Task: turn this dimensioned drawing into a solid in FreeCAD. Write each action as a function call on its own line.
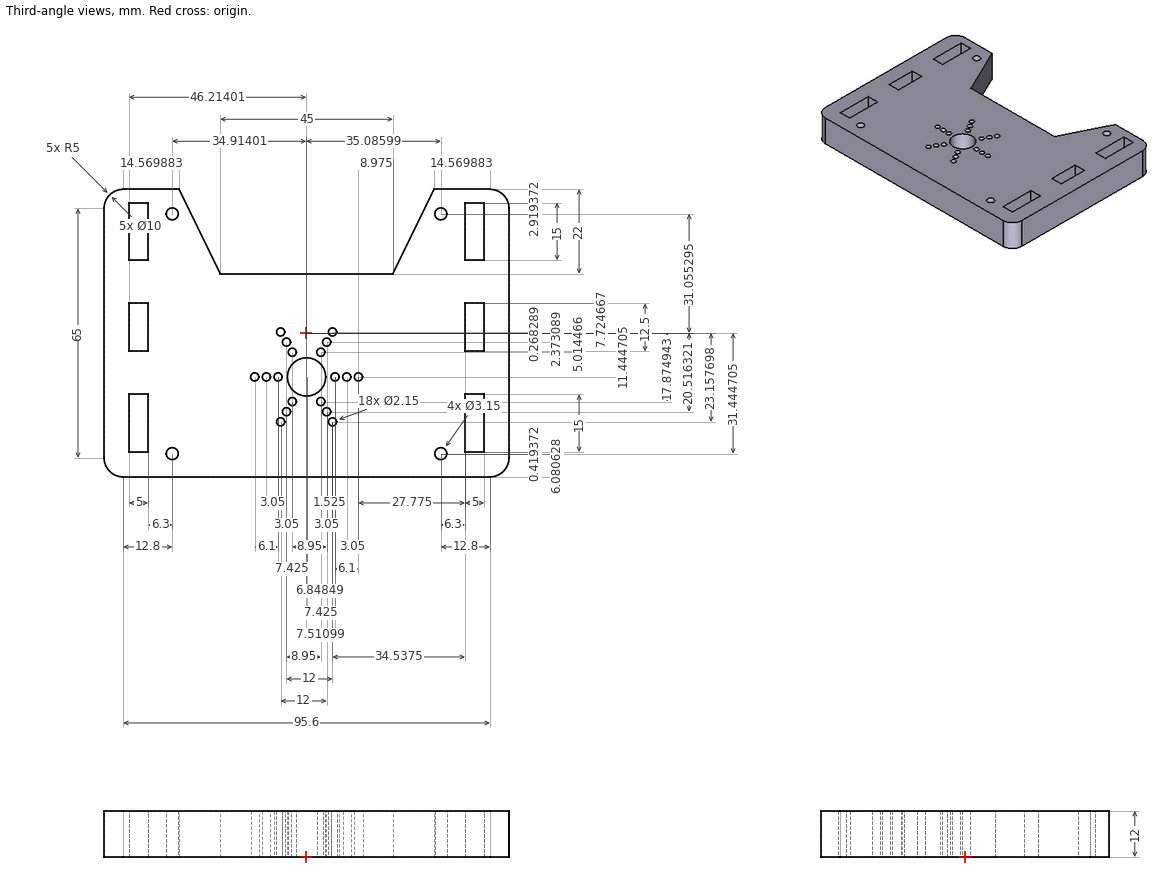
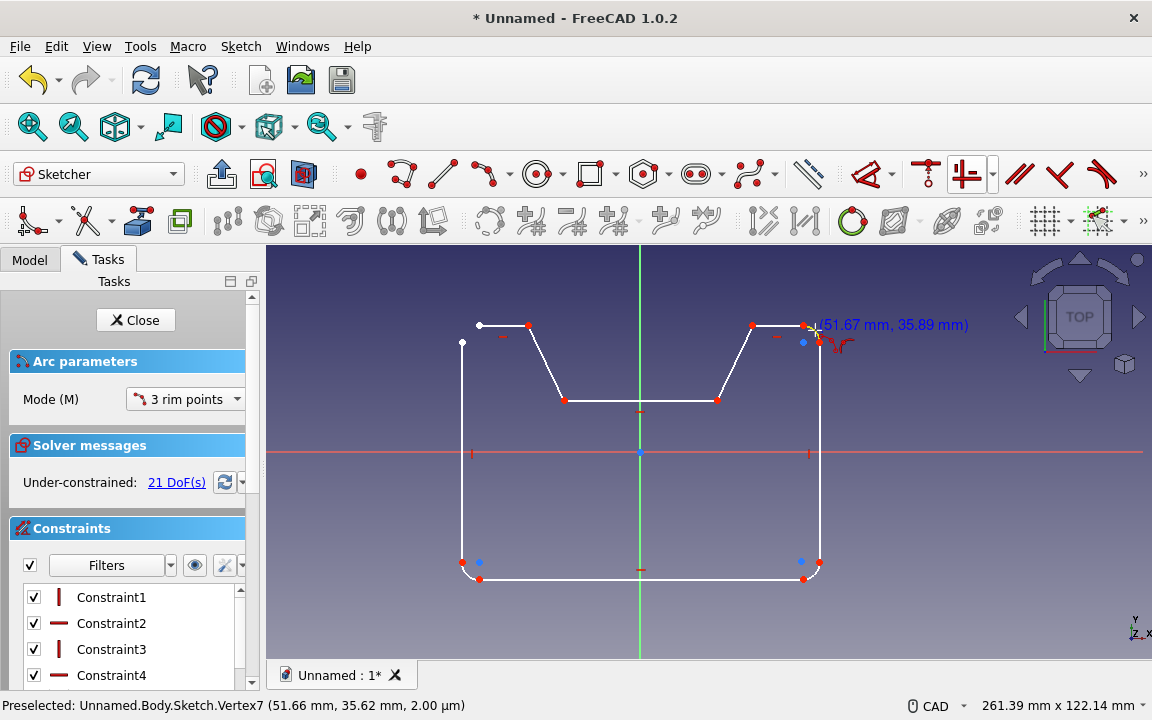
click(479, 326)
click(462, 343)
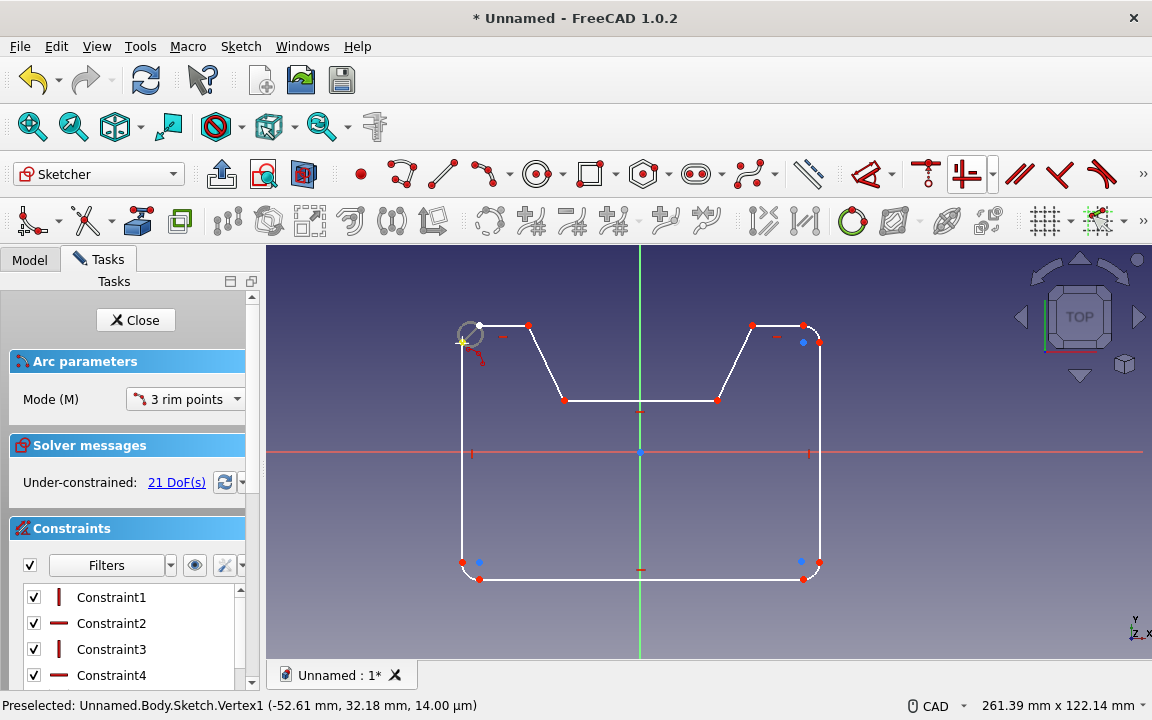
scroll(467, 330, up, 6)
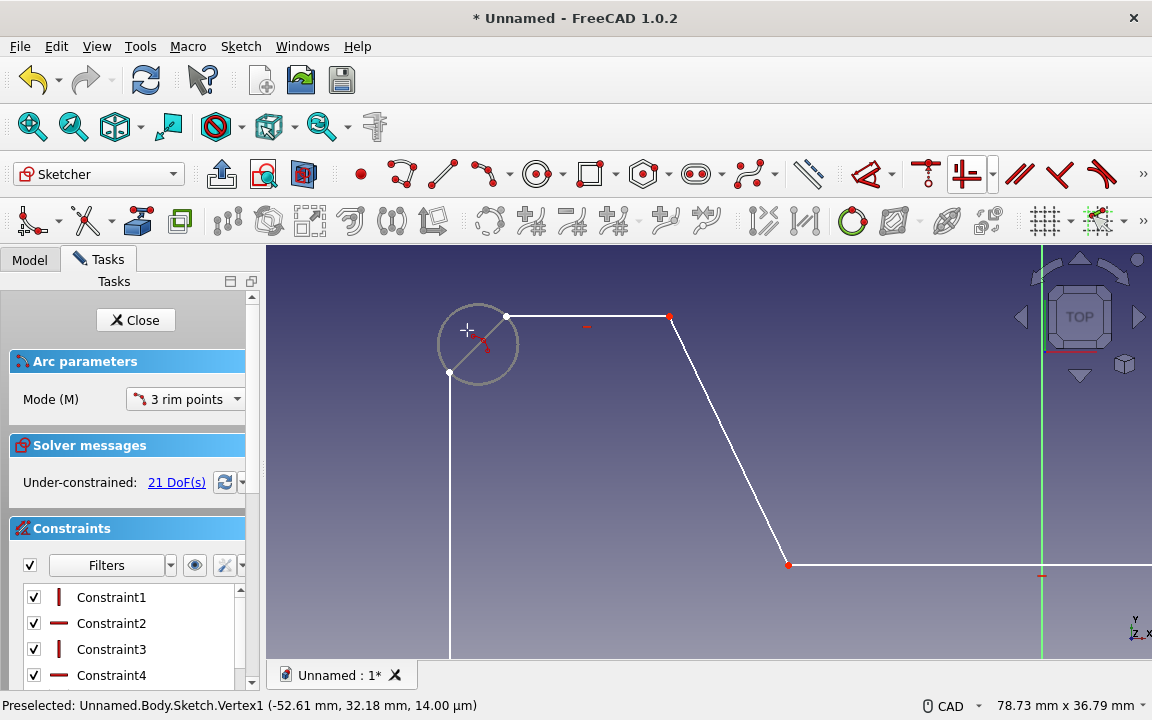
click(465, 330)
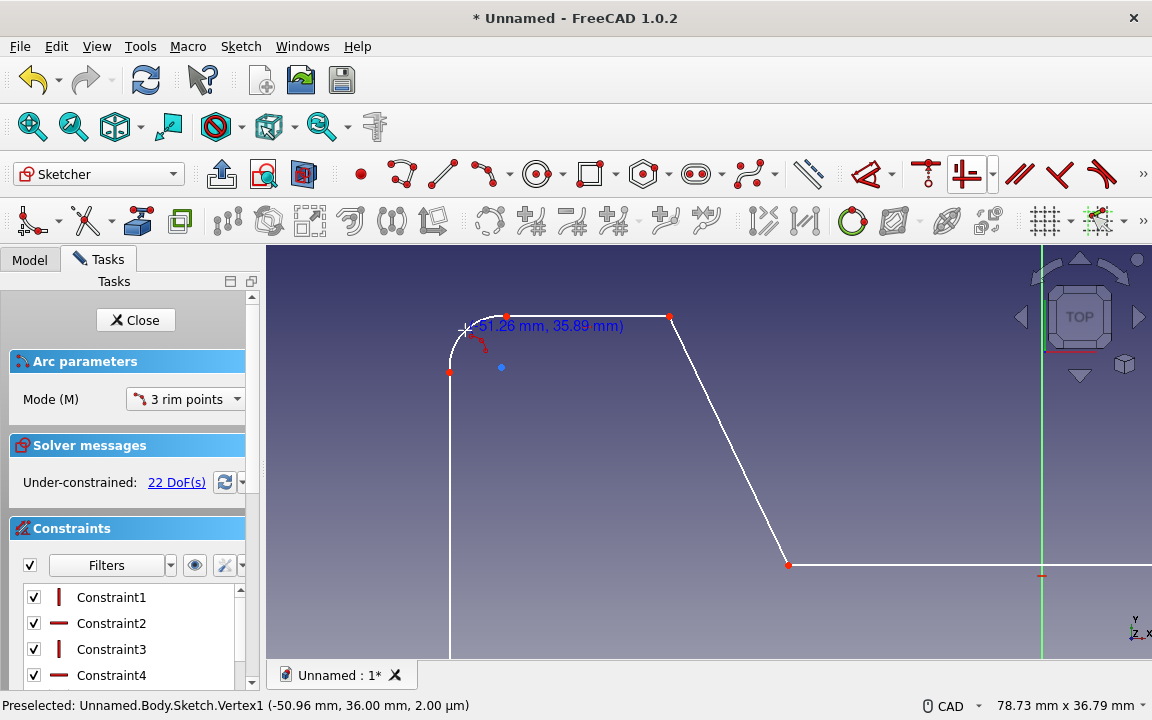
key(g)
key(r)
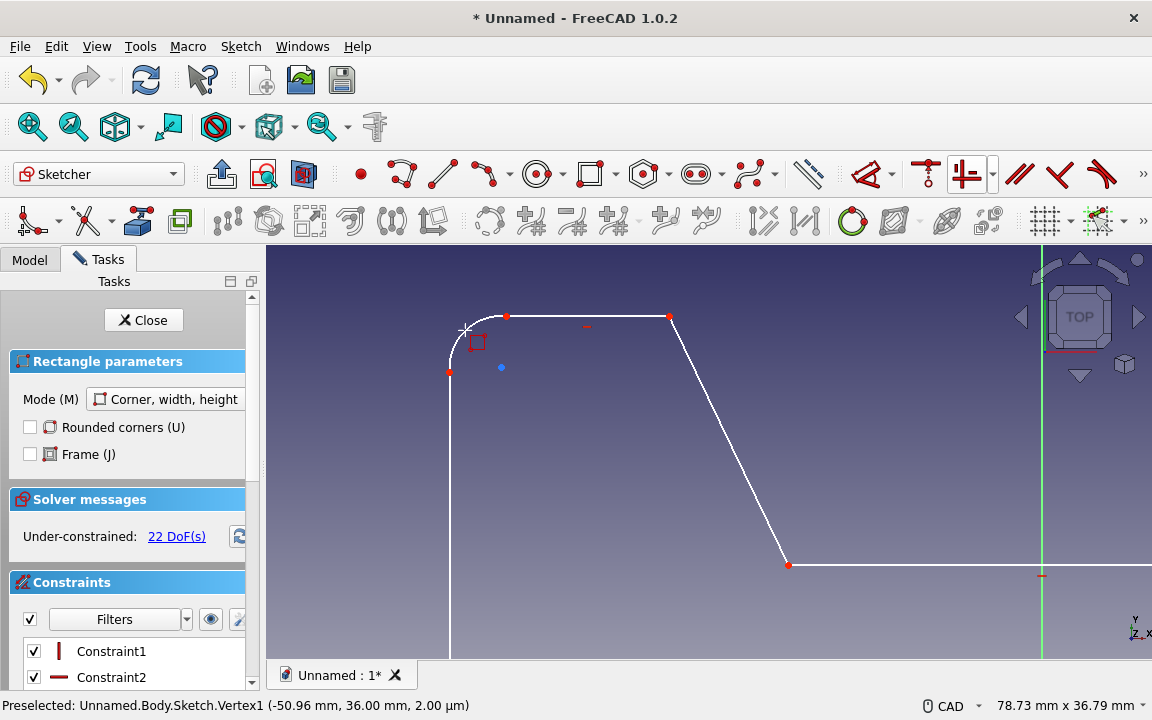
scroll(467, 330, down, 6)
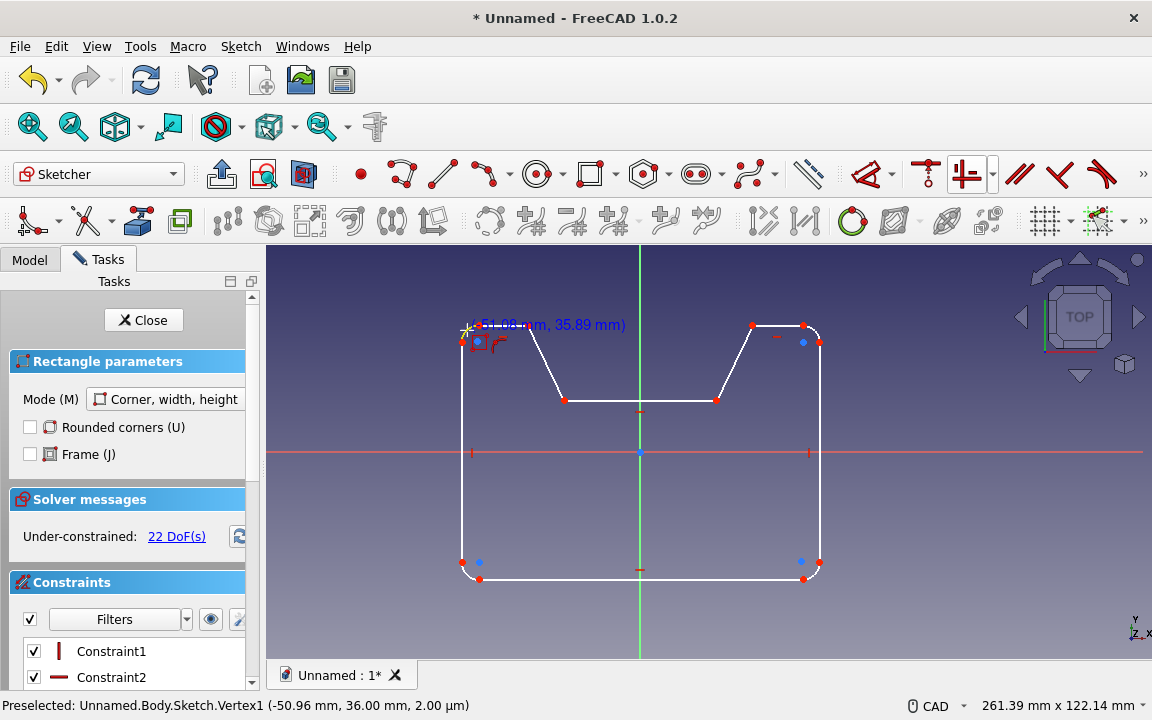
click(781, 506)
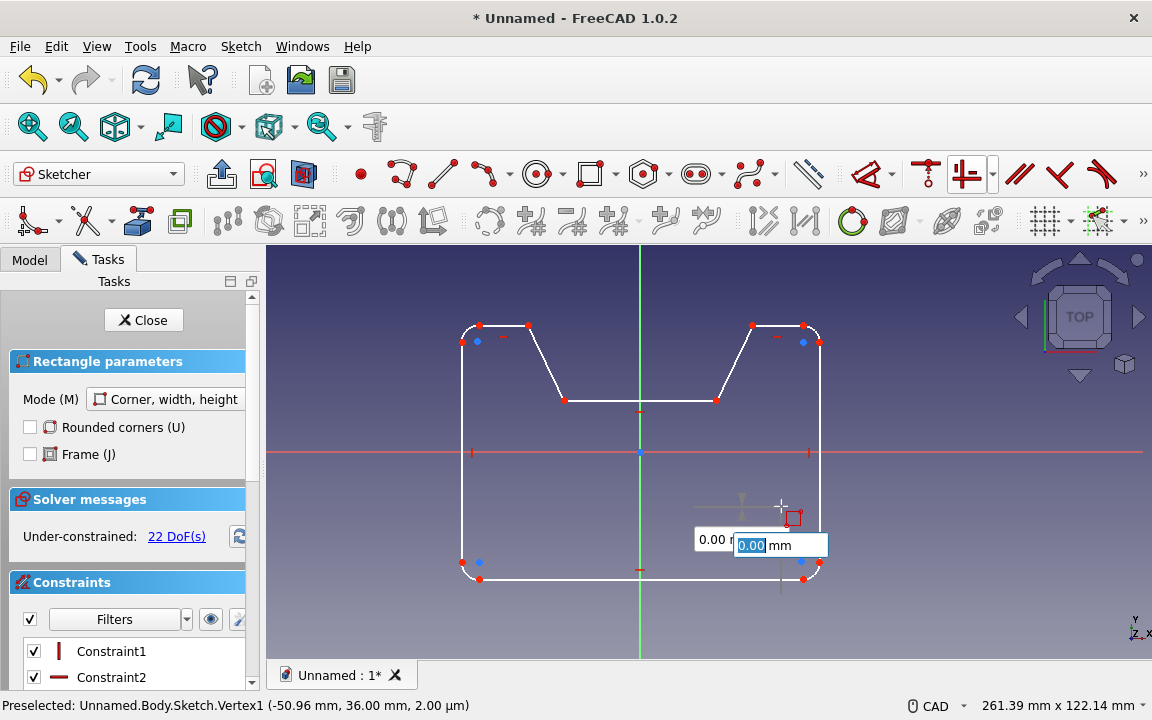
scroll(798, 557, up, 4)
move(796, 557)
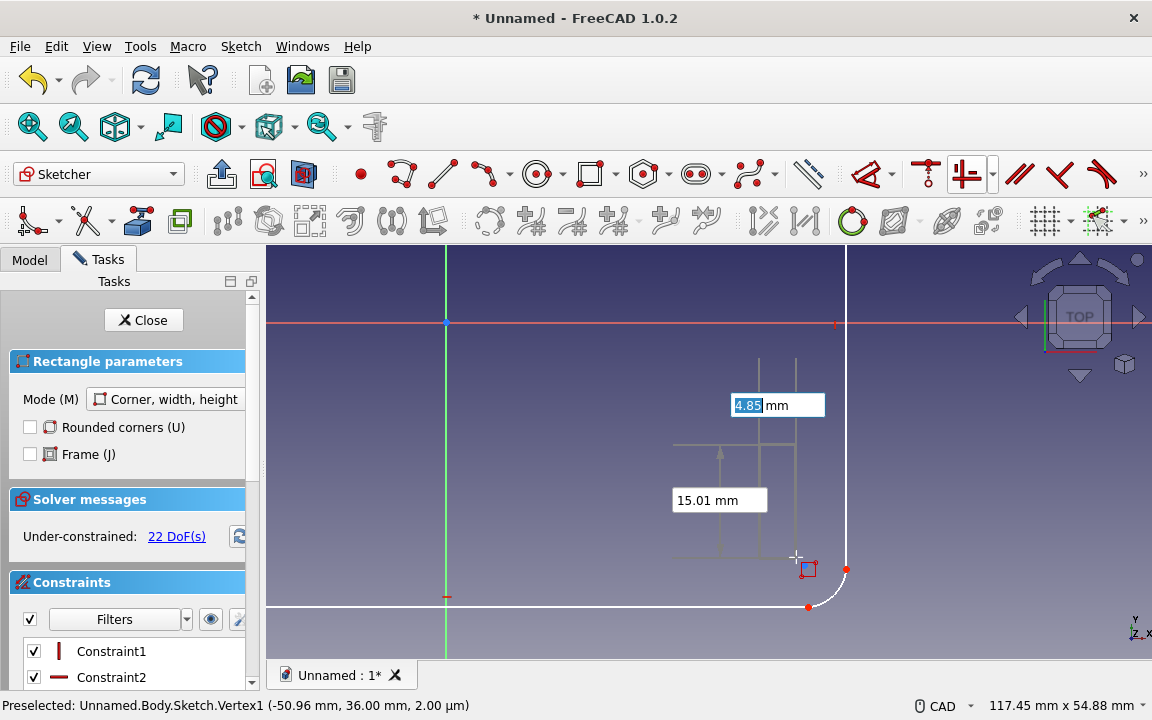
text(5)
key(Tab)
text(15)
key(Return)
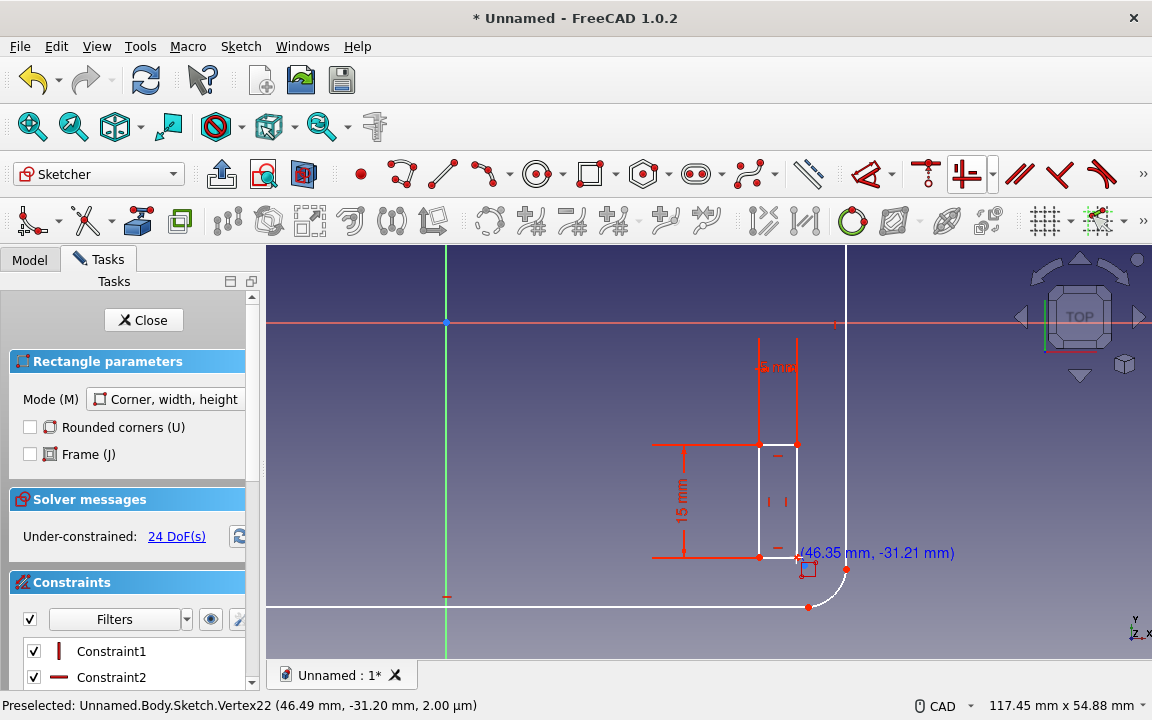
scroll(798, 557, down, 4)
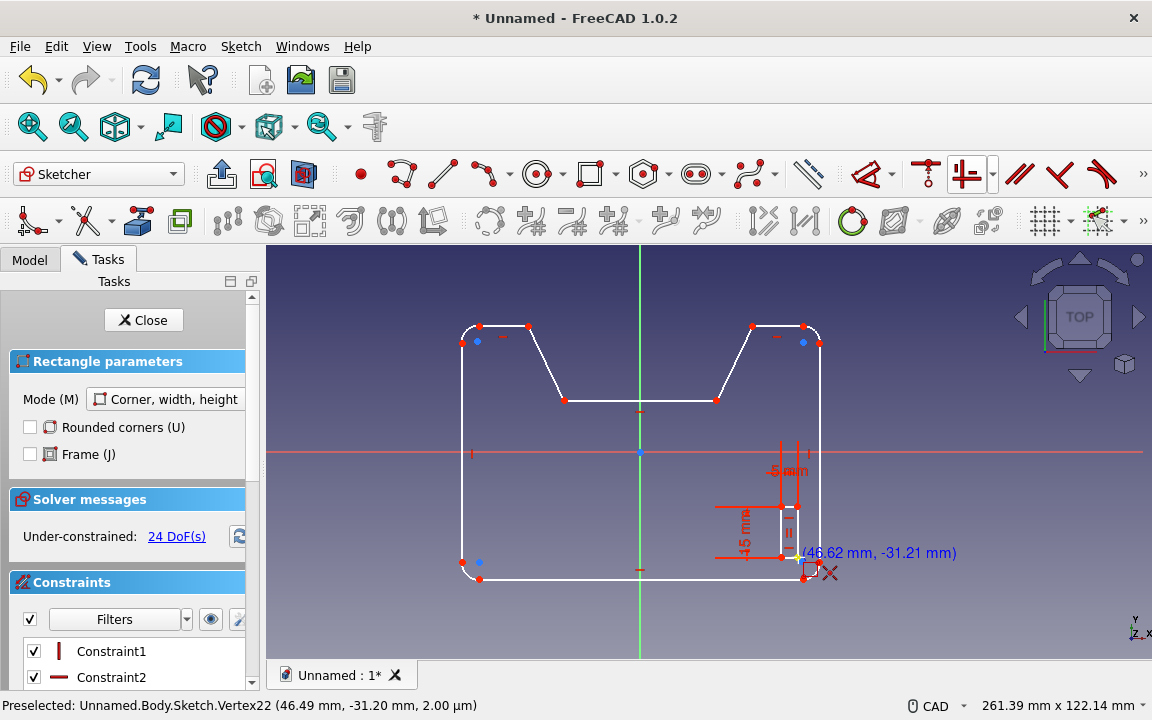
click(484, 506)
move(501, 557)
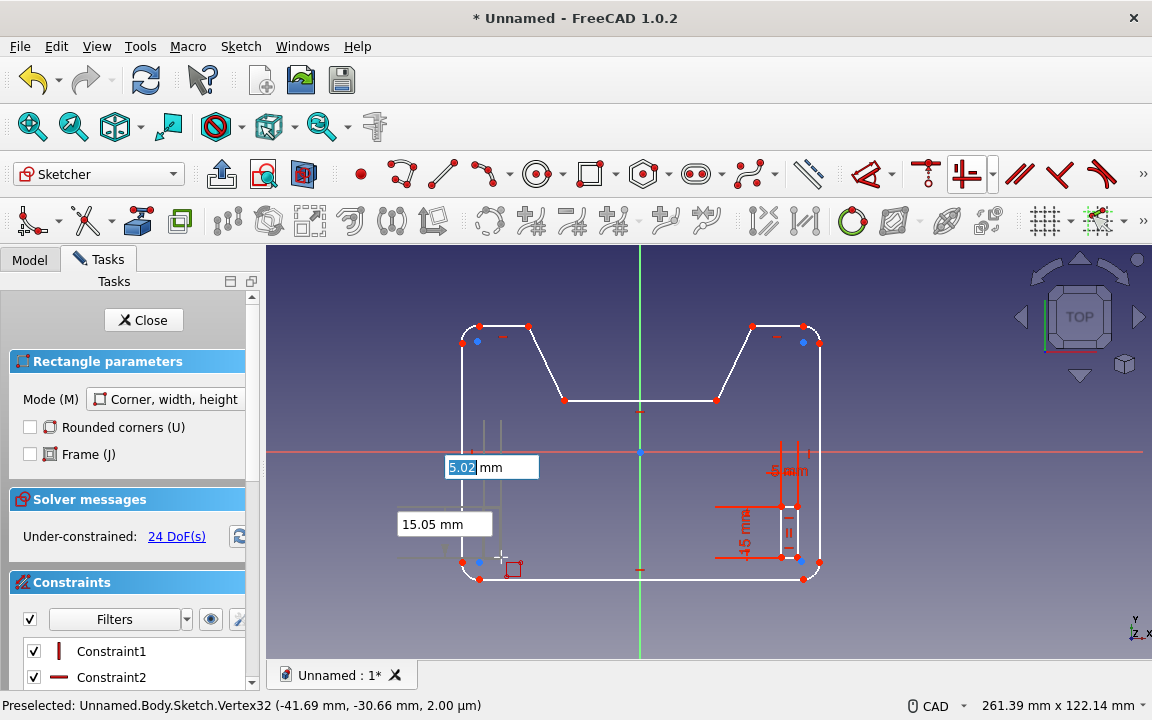
text(5)
key(Tab)
text(15)
key(Return)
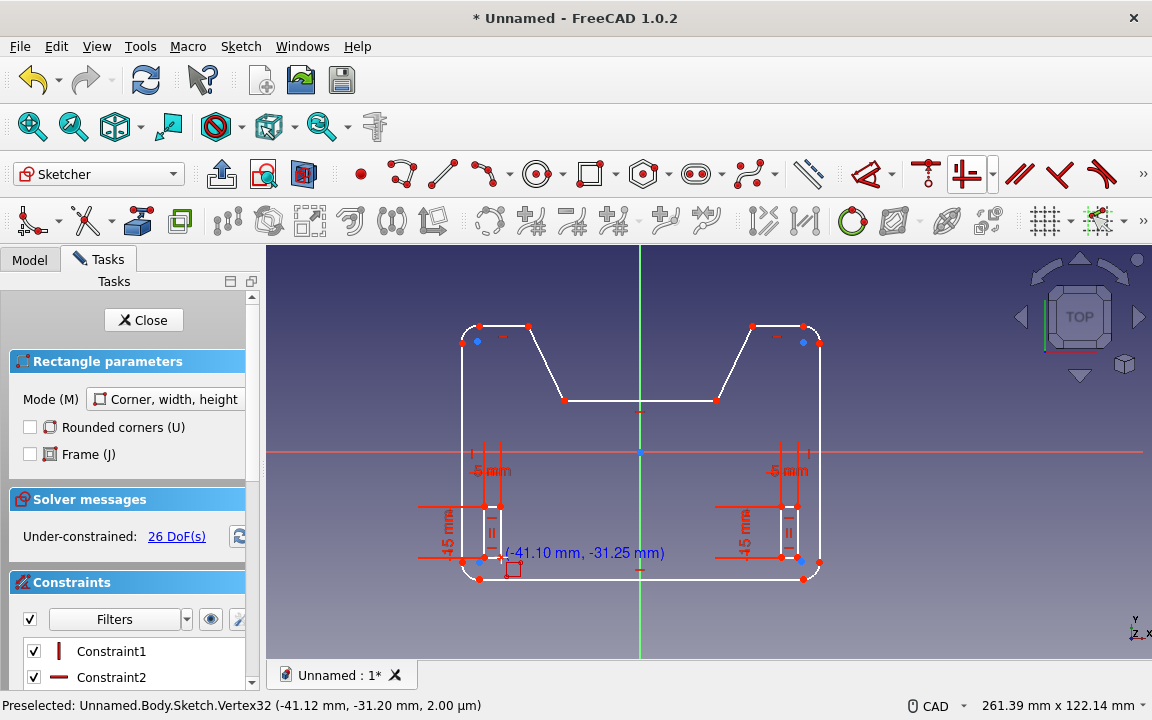
click(781, 426)
move(798, 468)